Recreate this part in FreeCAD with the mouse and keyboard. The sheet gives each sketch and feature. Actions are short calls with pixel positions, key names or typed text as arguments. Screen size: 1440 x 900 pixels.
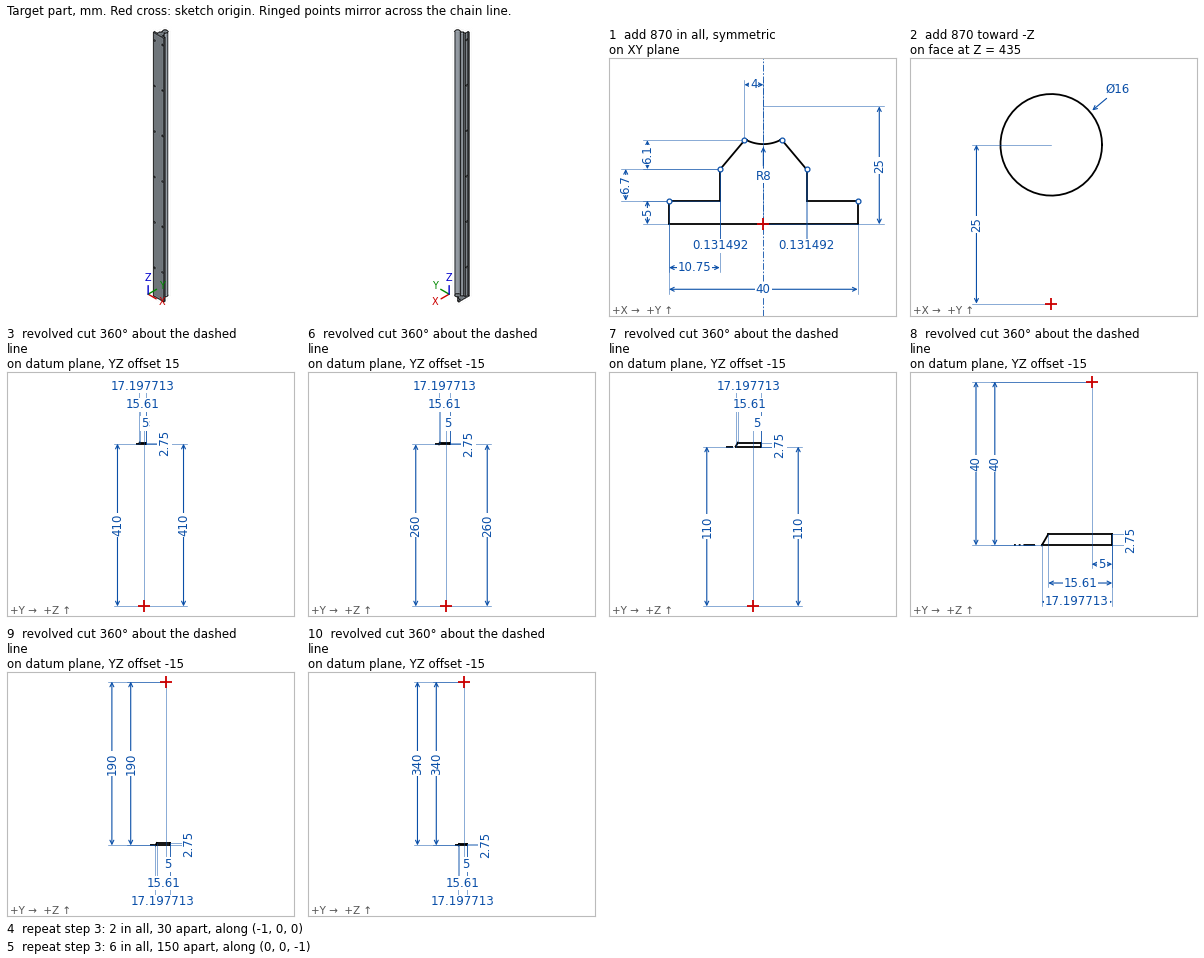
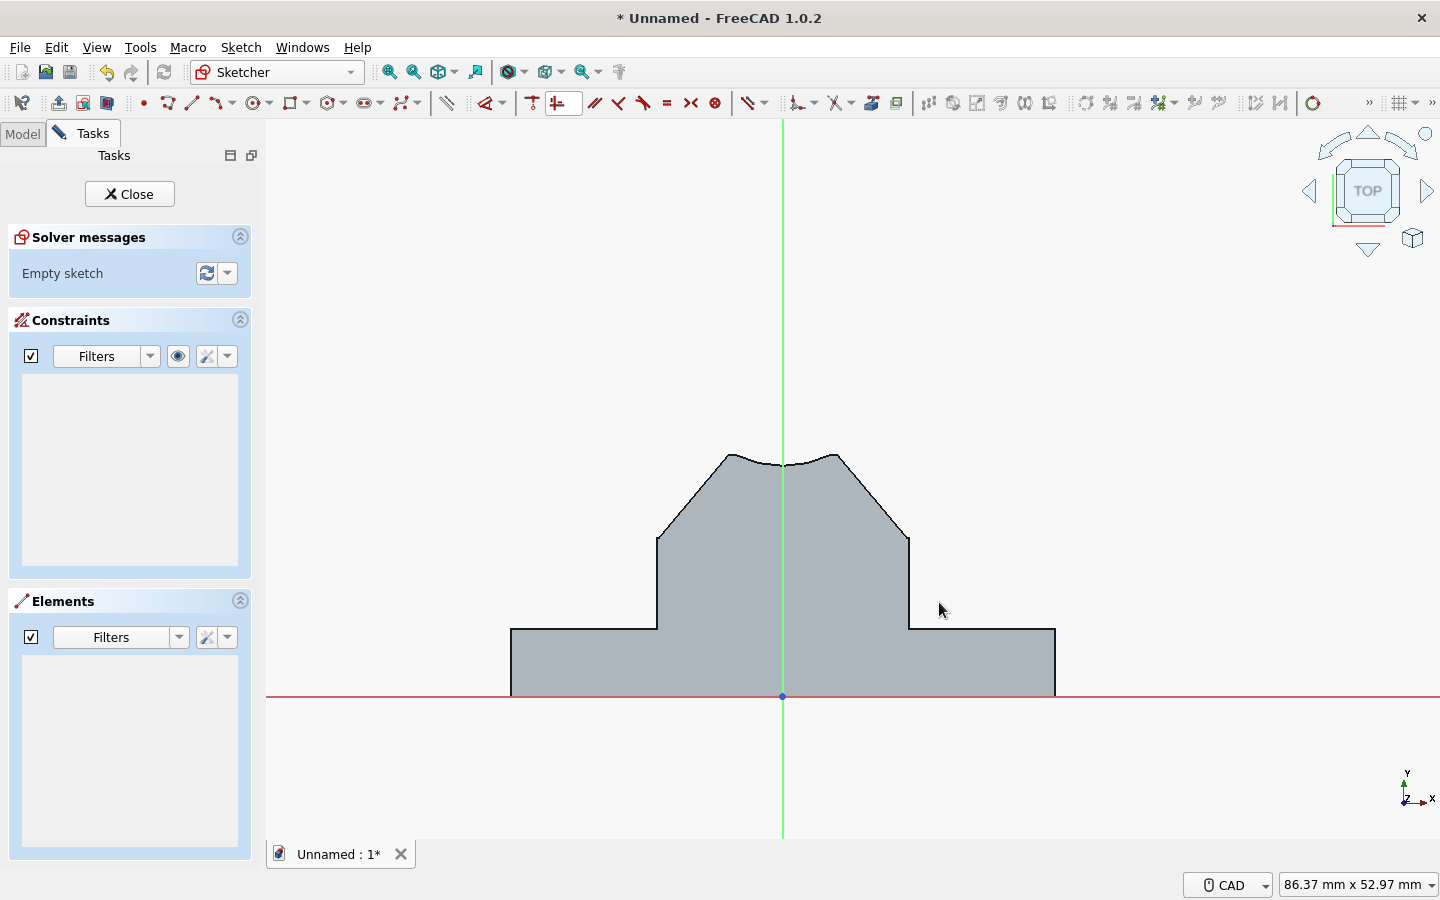
click(254, 104)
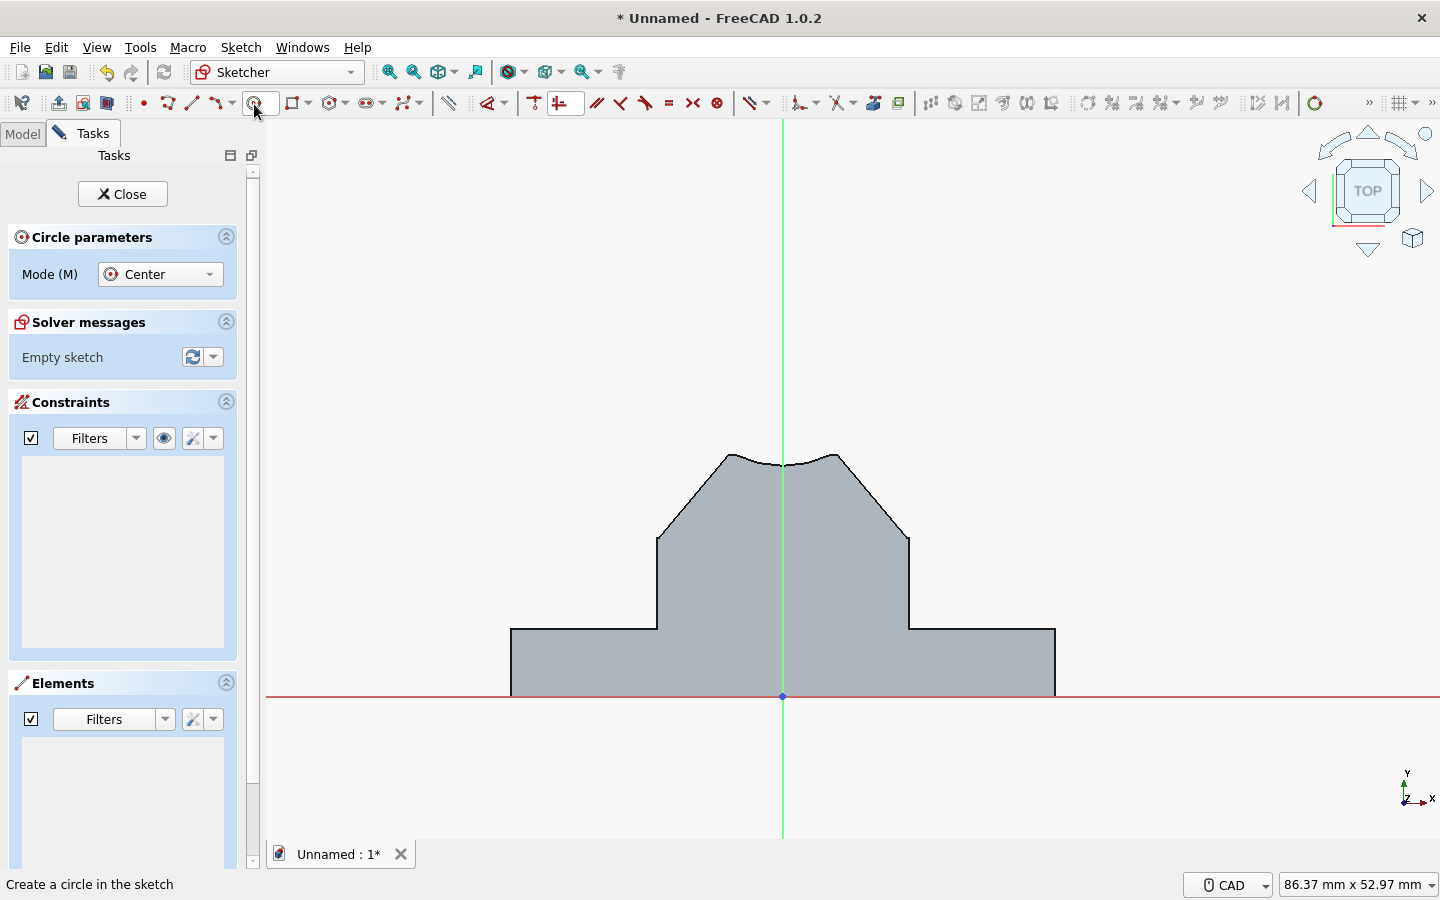
click(783, 357)
move(860, 280)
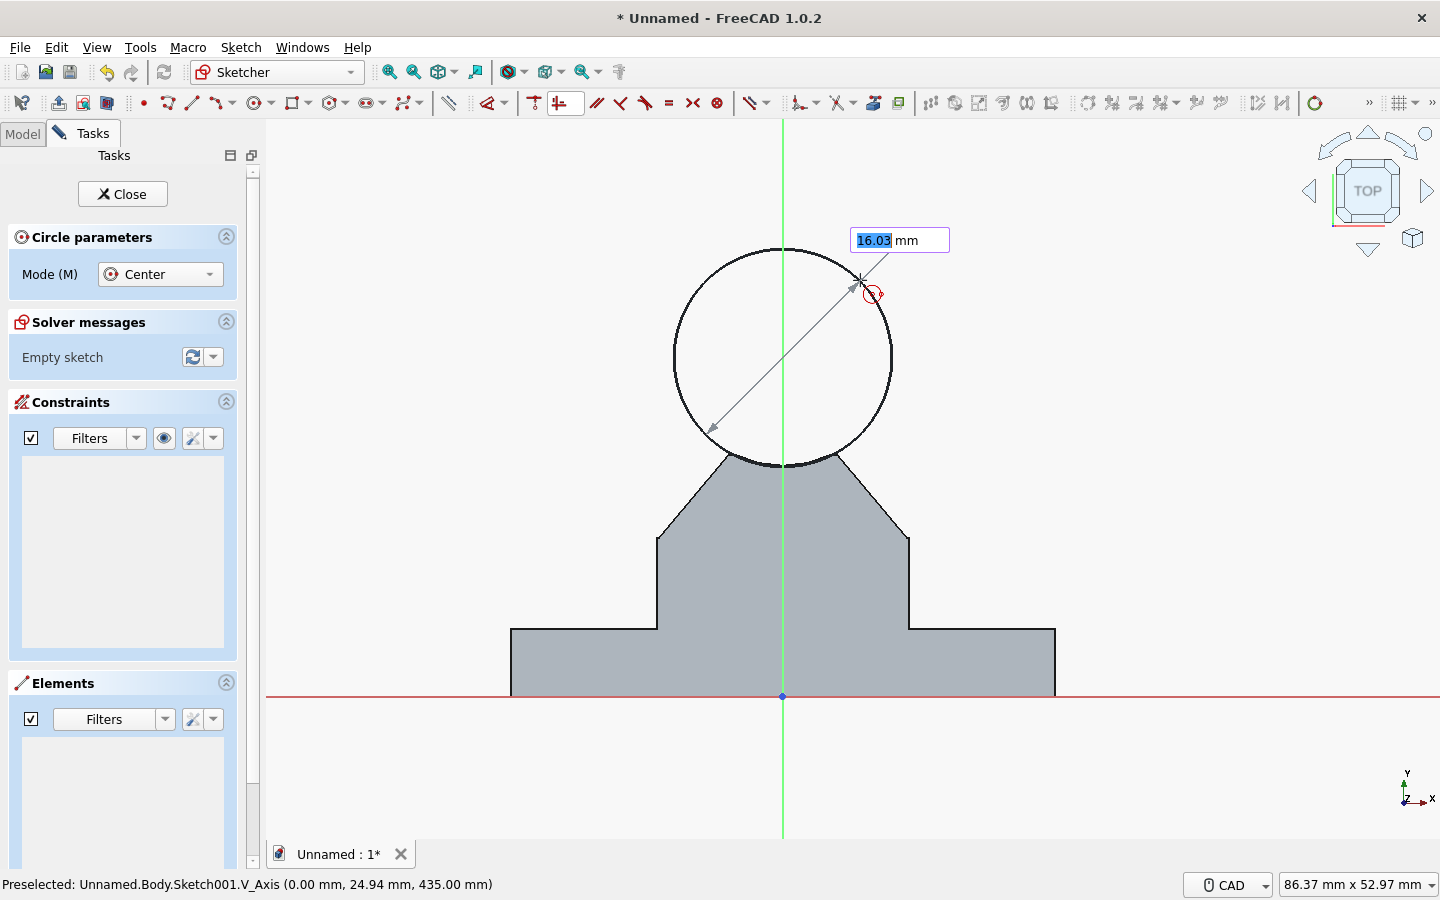
text(16)
key(Return)
key(Escape)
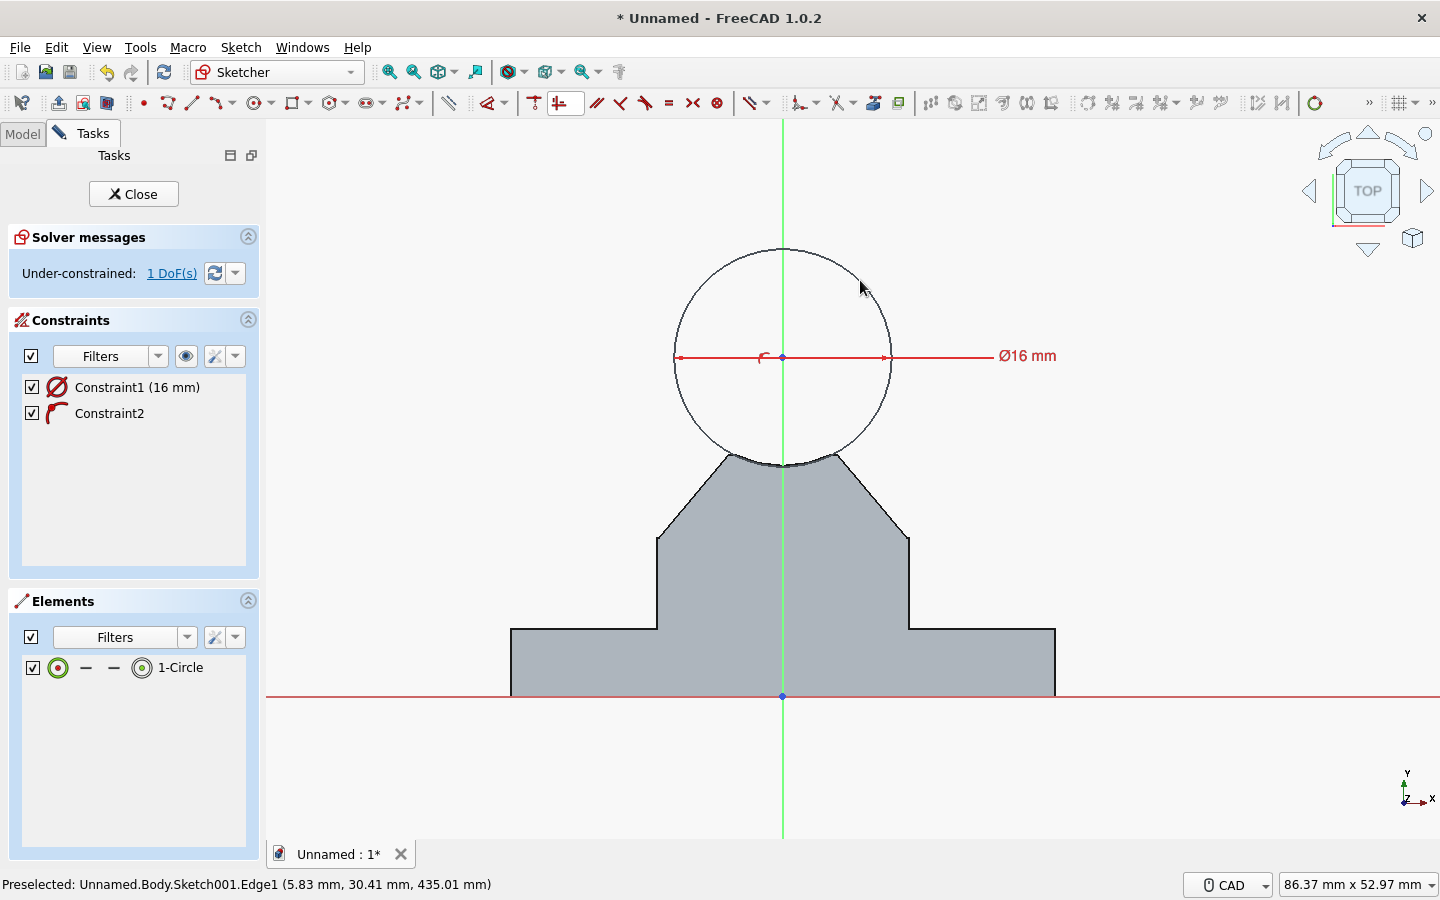
click(488, 104)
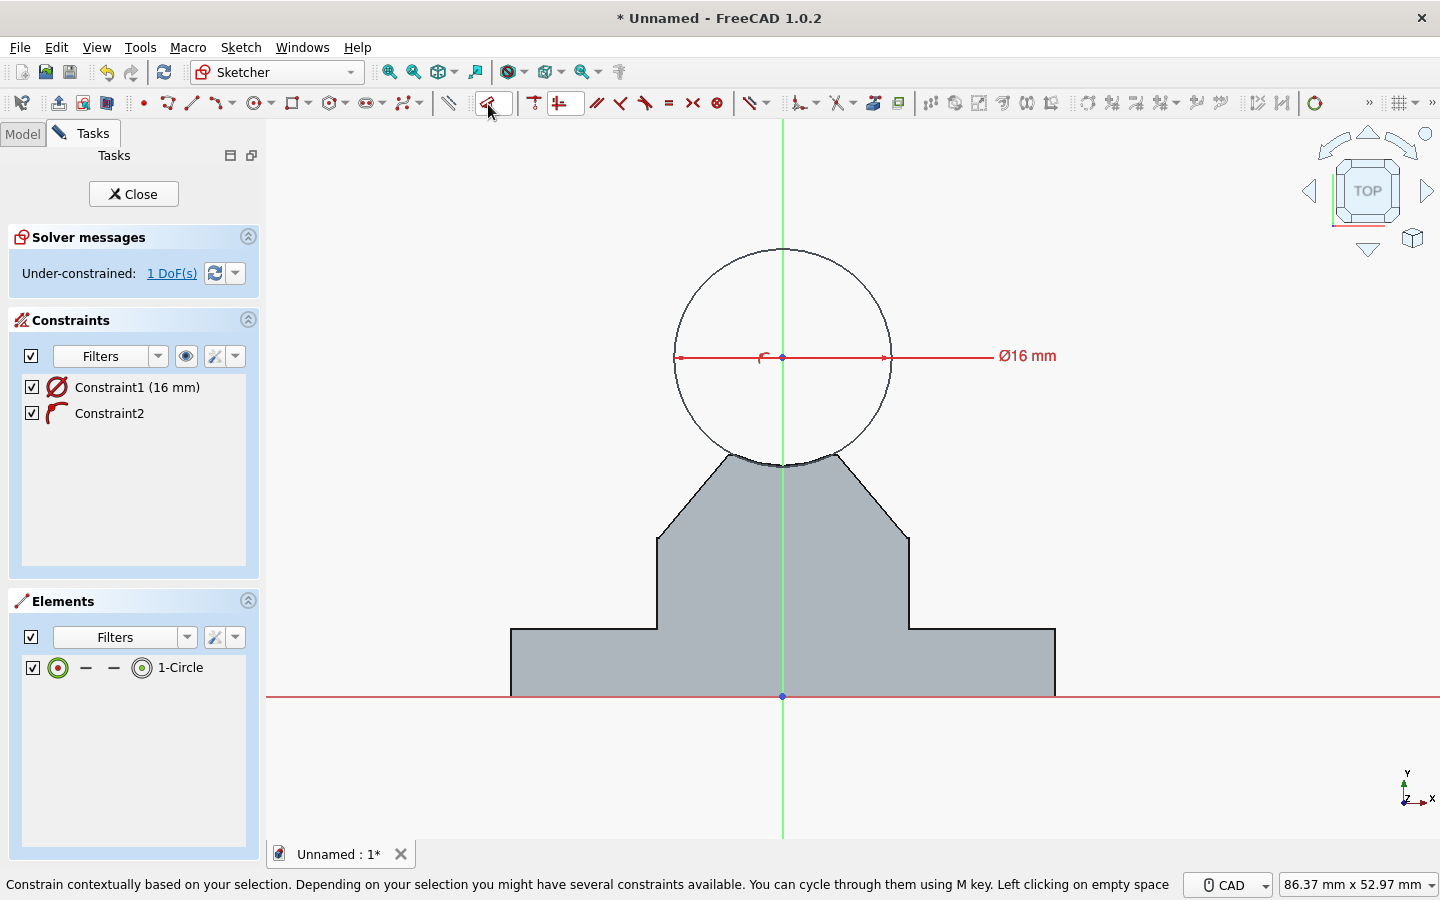
click(783, 358)
click(817, 527)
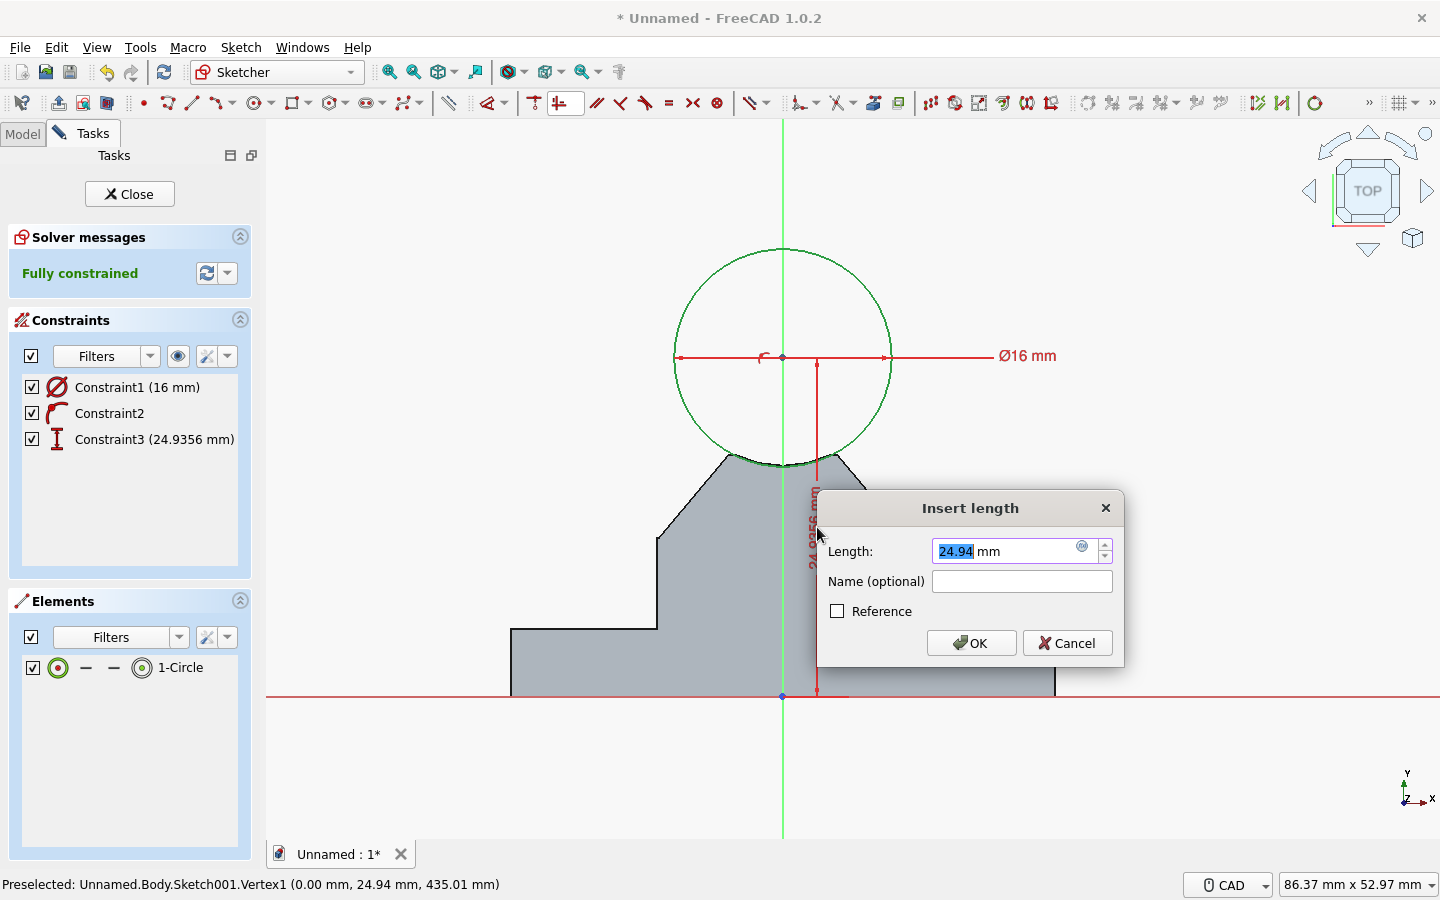
text(25)
key(Return)
key(Escape)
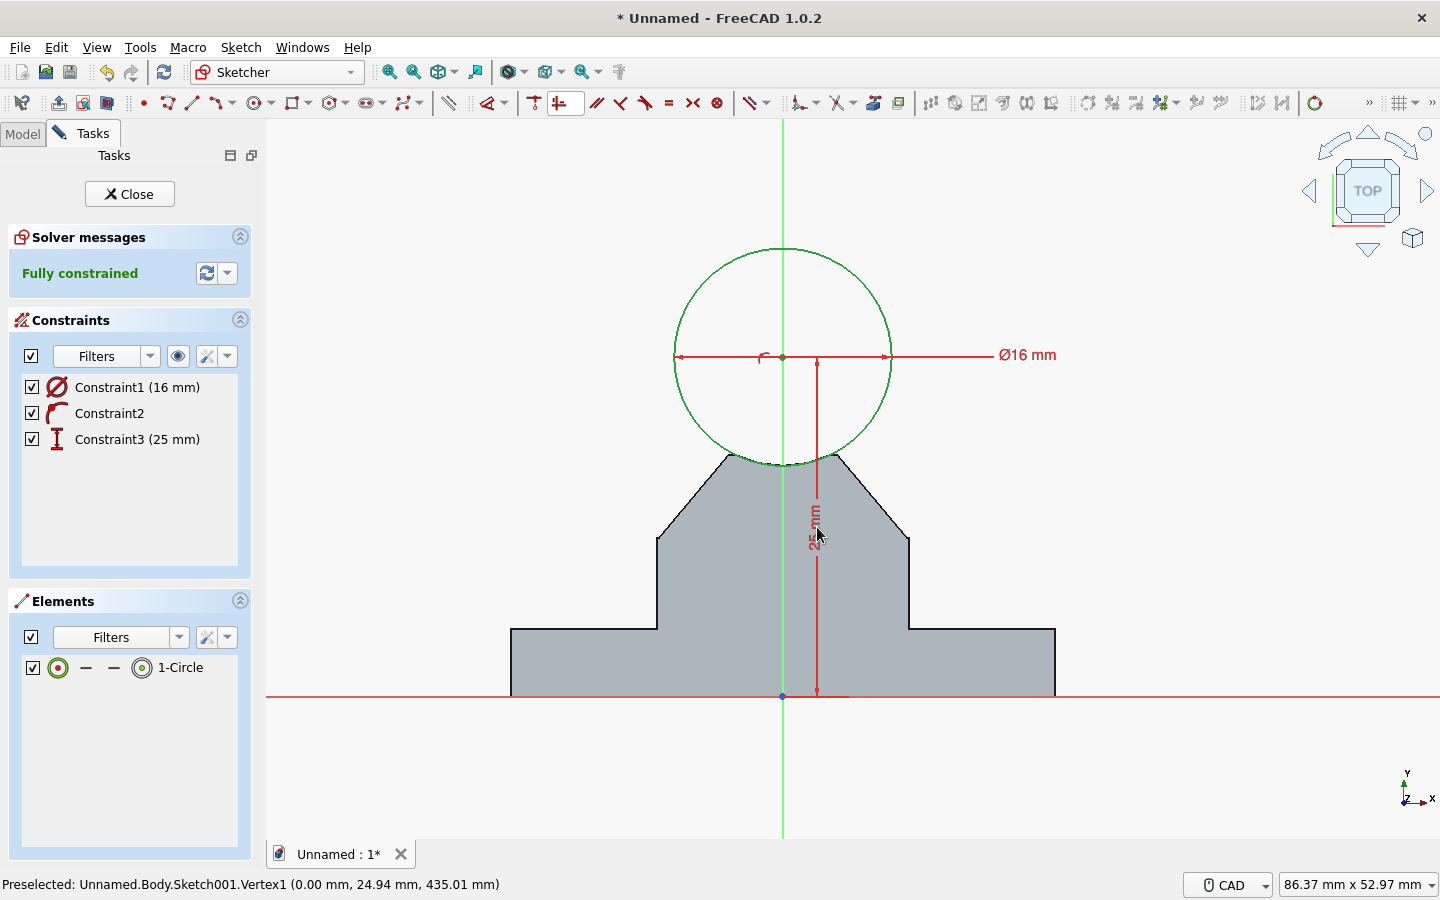
click(130, 194)